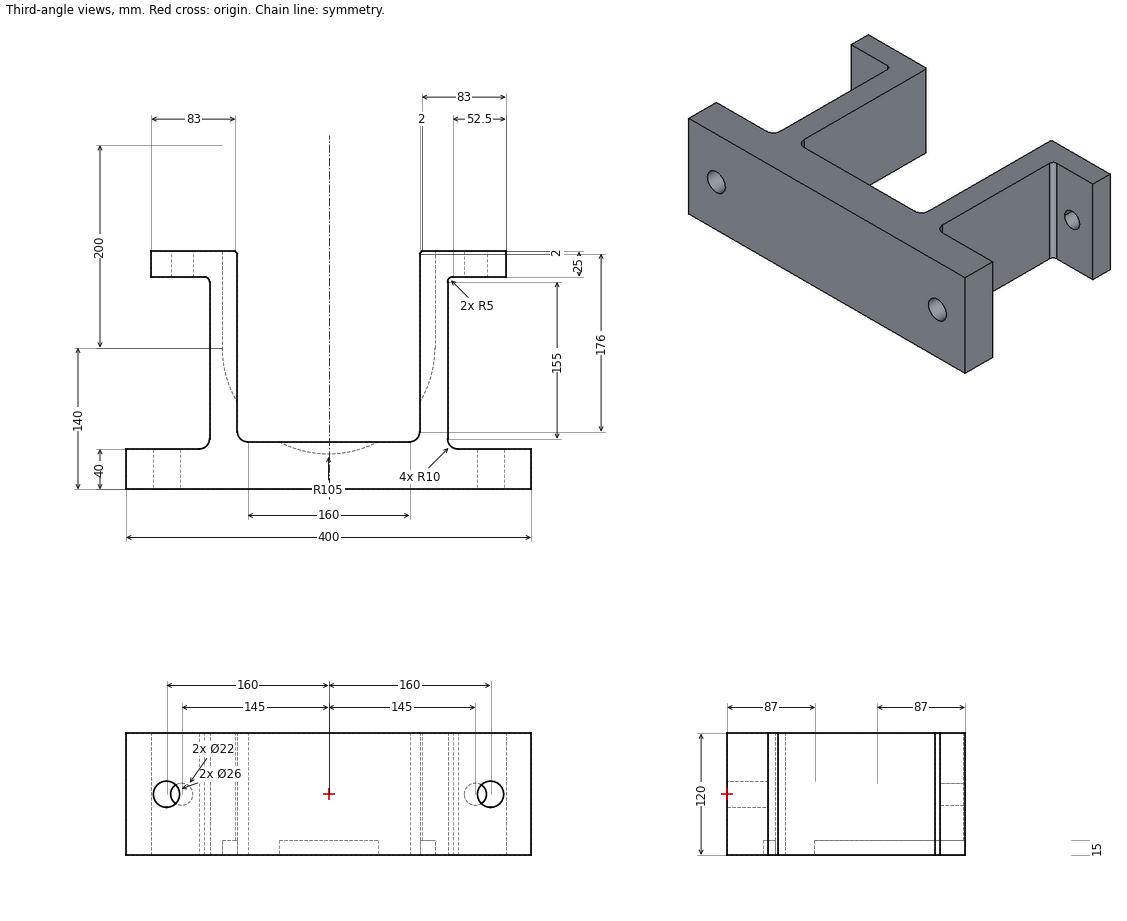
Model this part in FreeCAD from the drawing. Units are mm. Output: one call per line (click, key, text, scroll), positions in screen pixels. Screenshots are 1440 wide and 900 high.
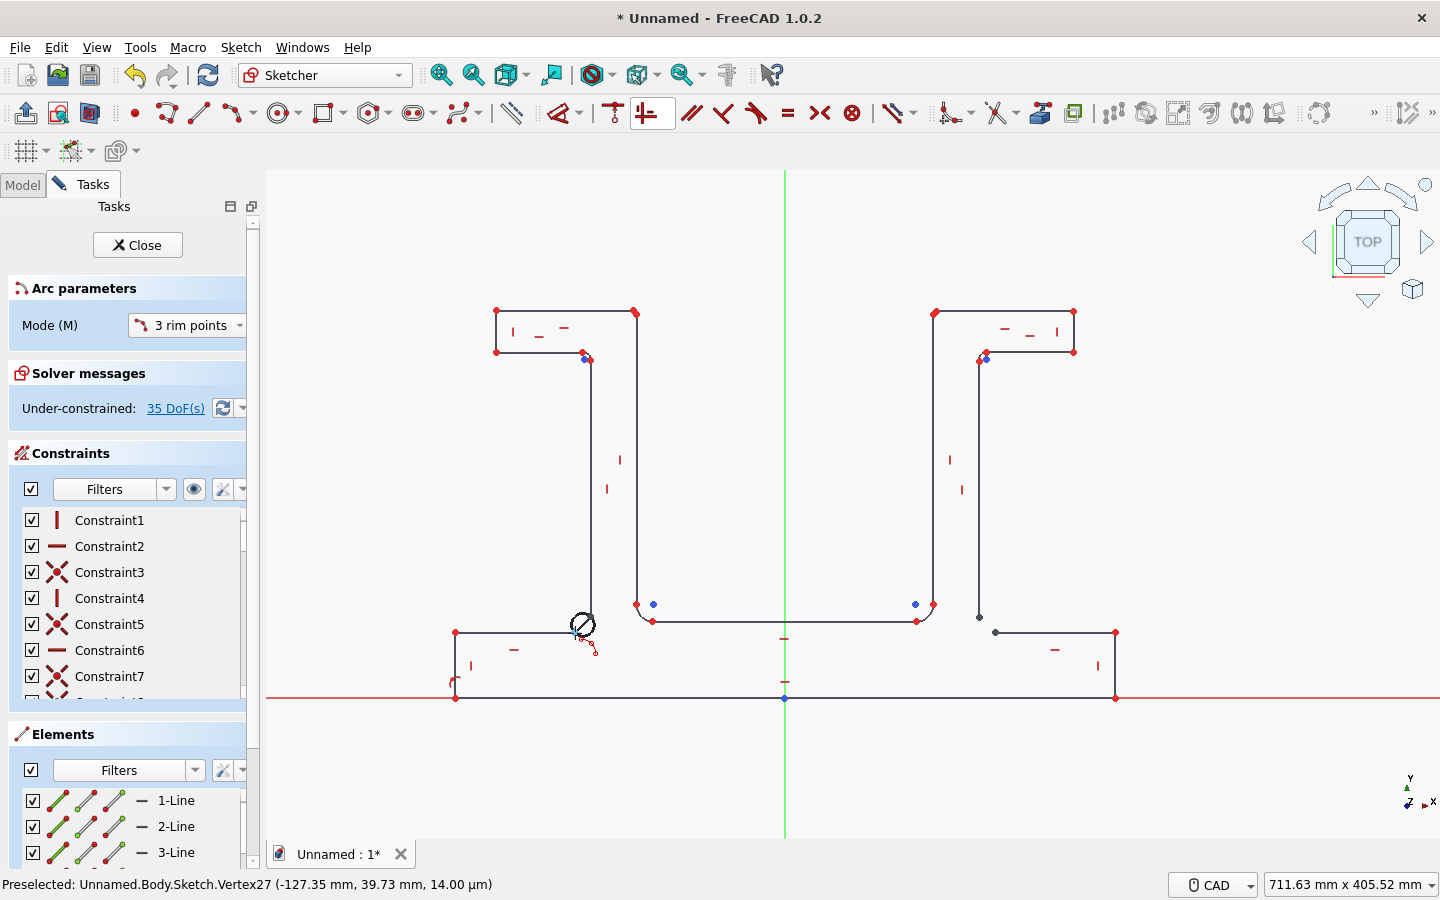
scroll(586, 628, up, 6)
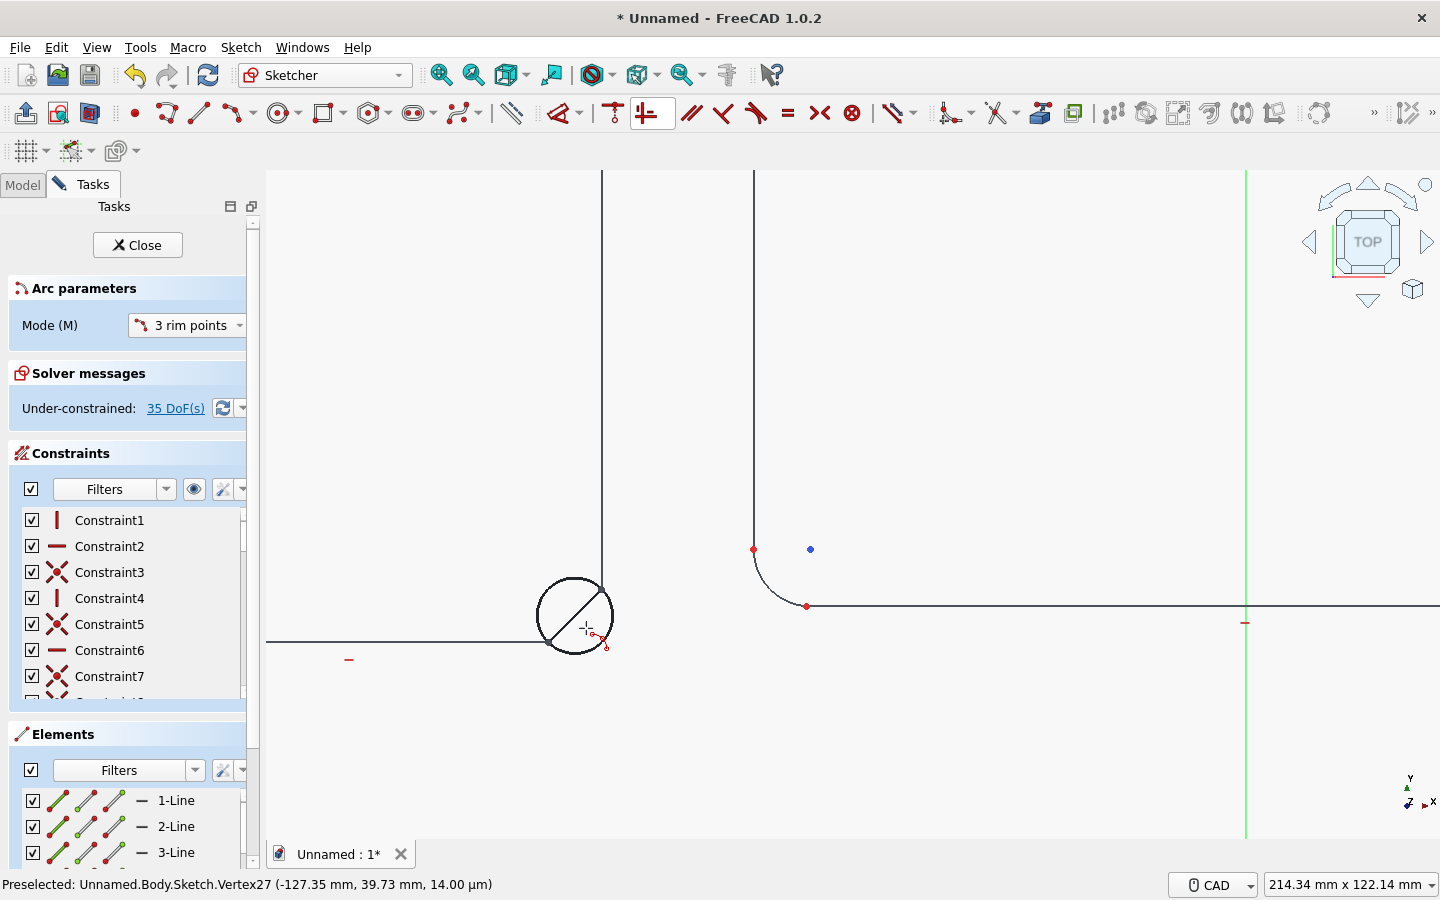
click(586, 625)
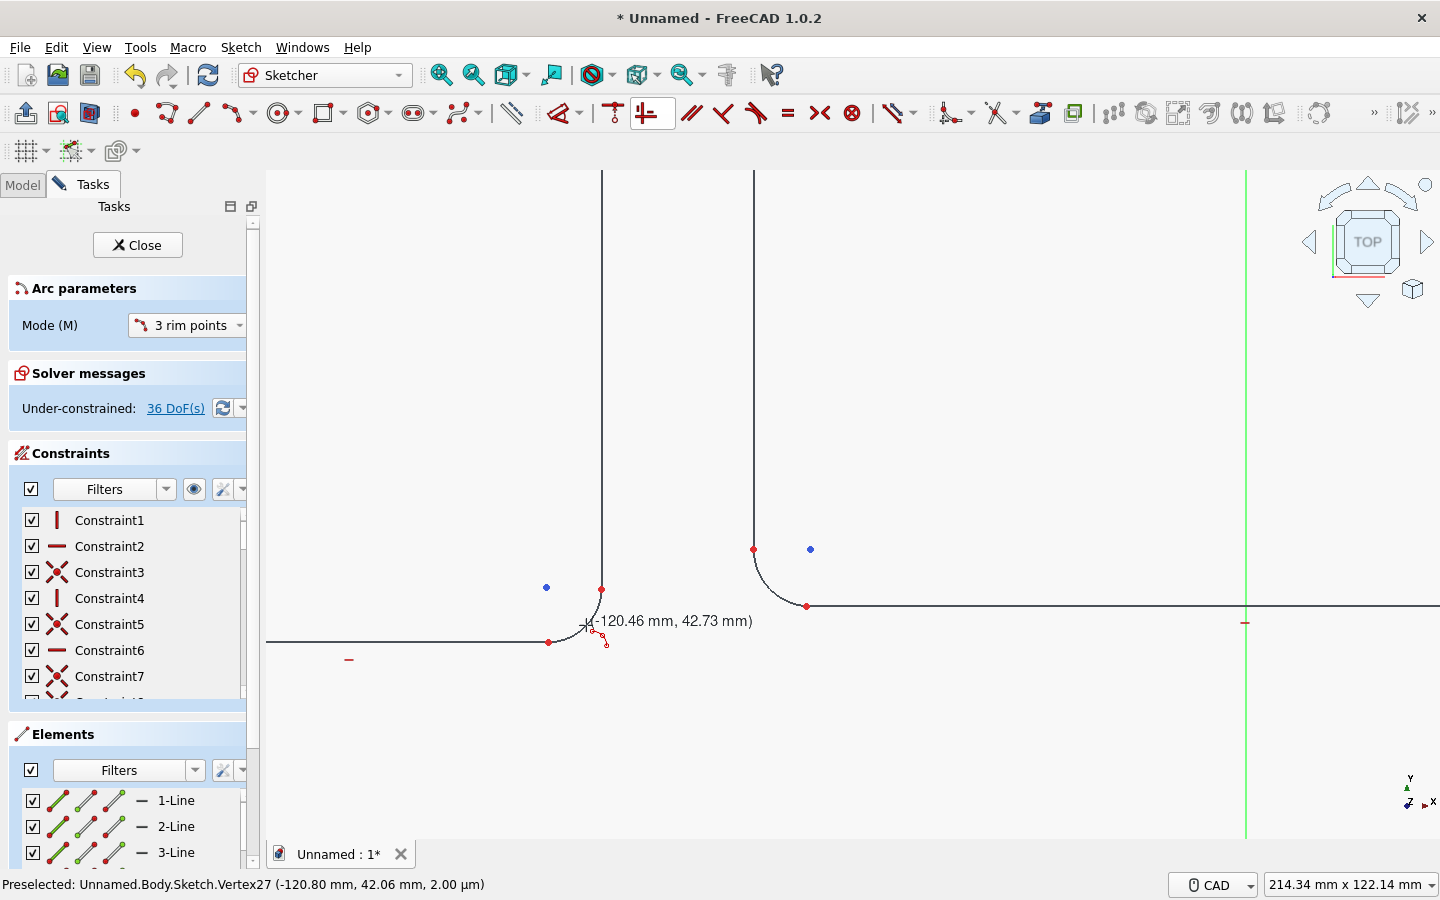
scroll(586, 629, down, 6)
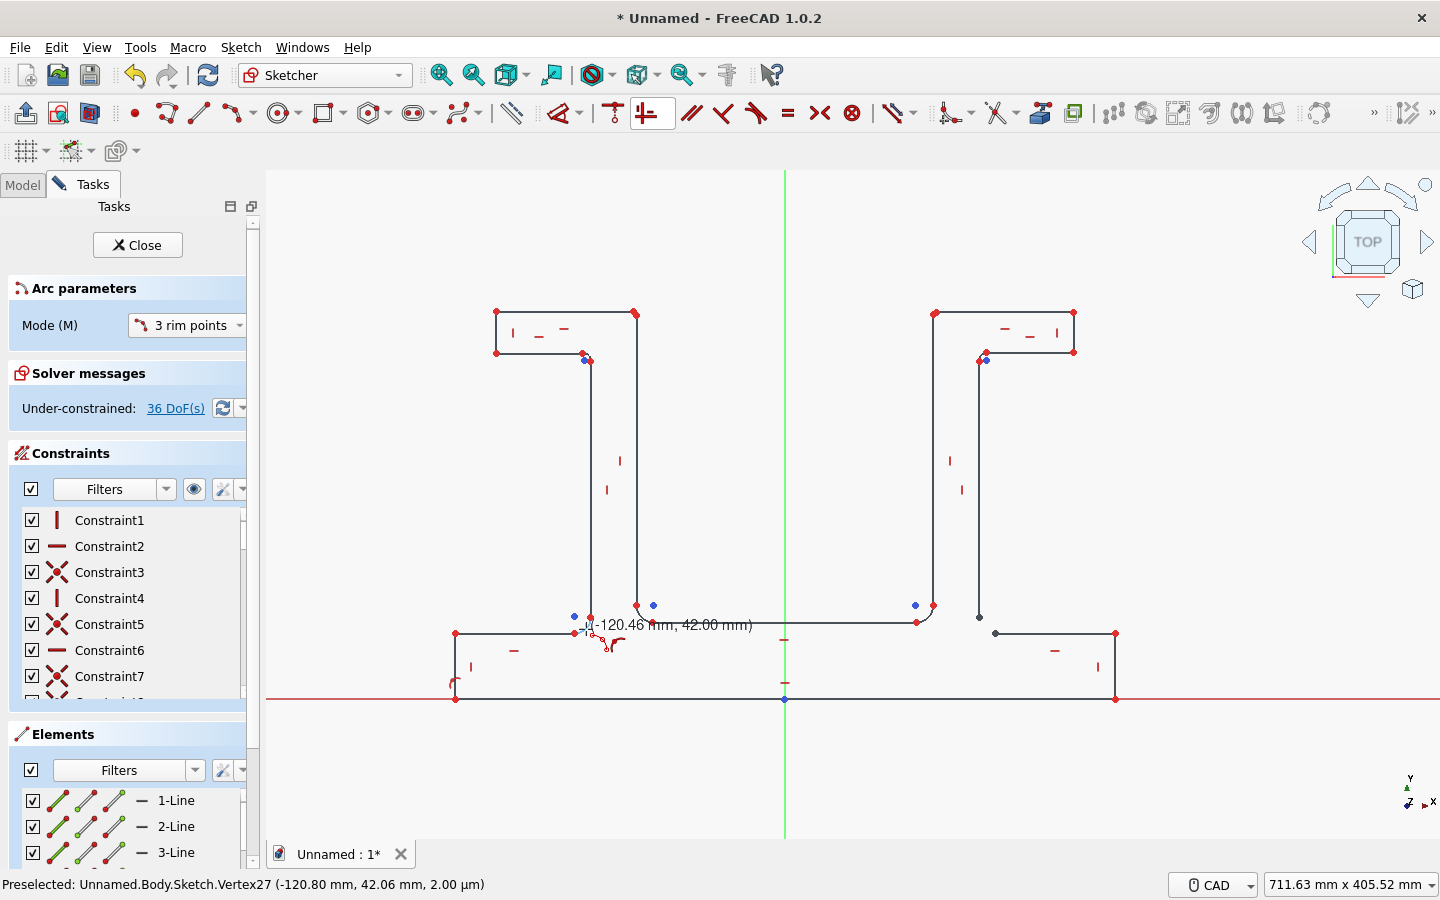
click(995, 634)
click(979, 618)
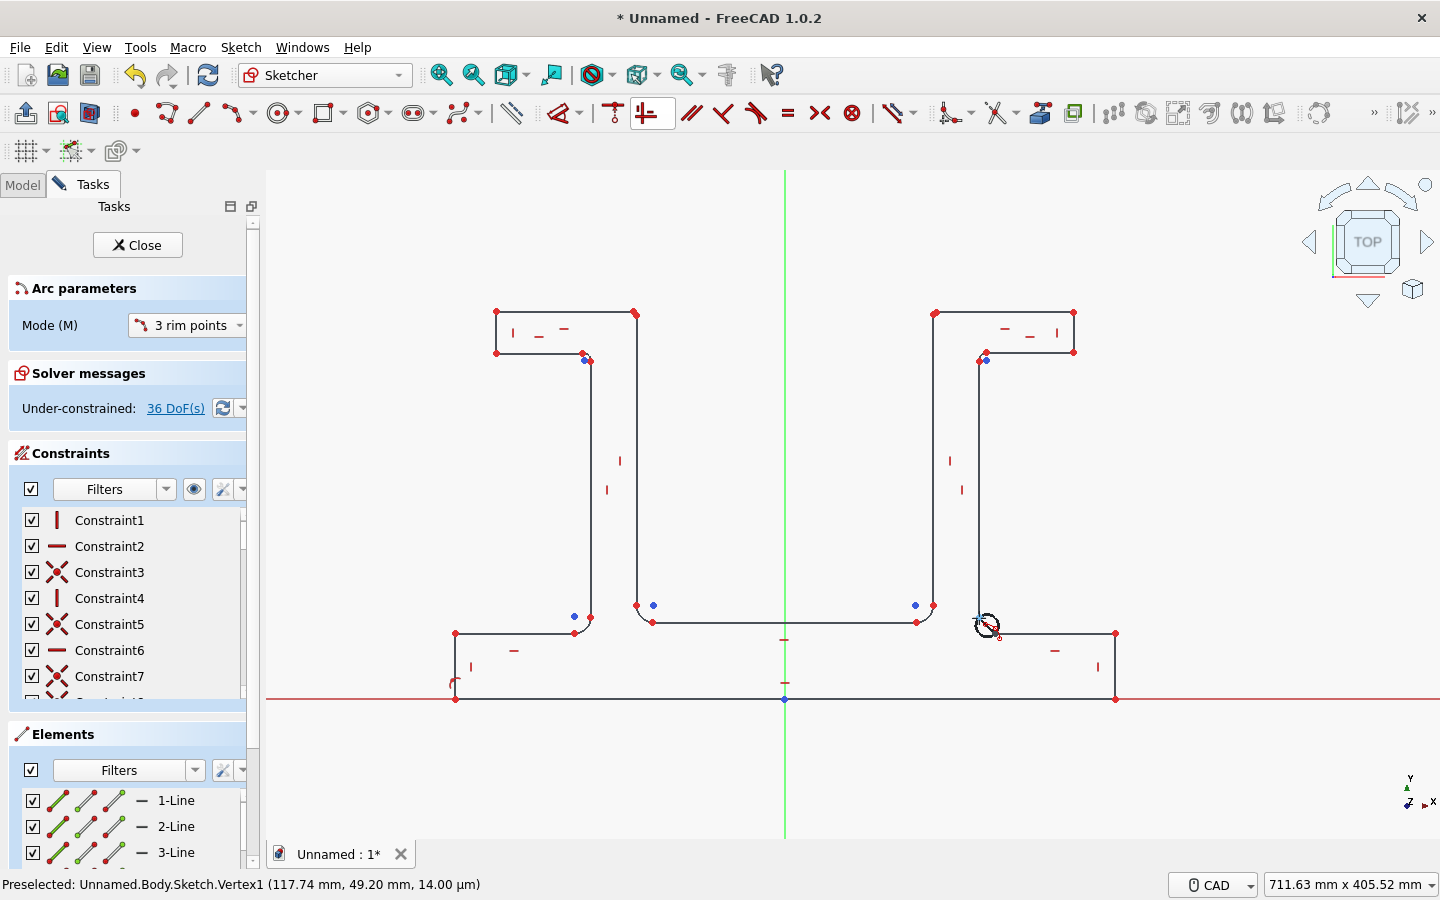
scroll(984, 628, up, 6)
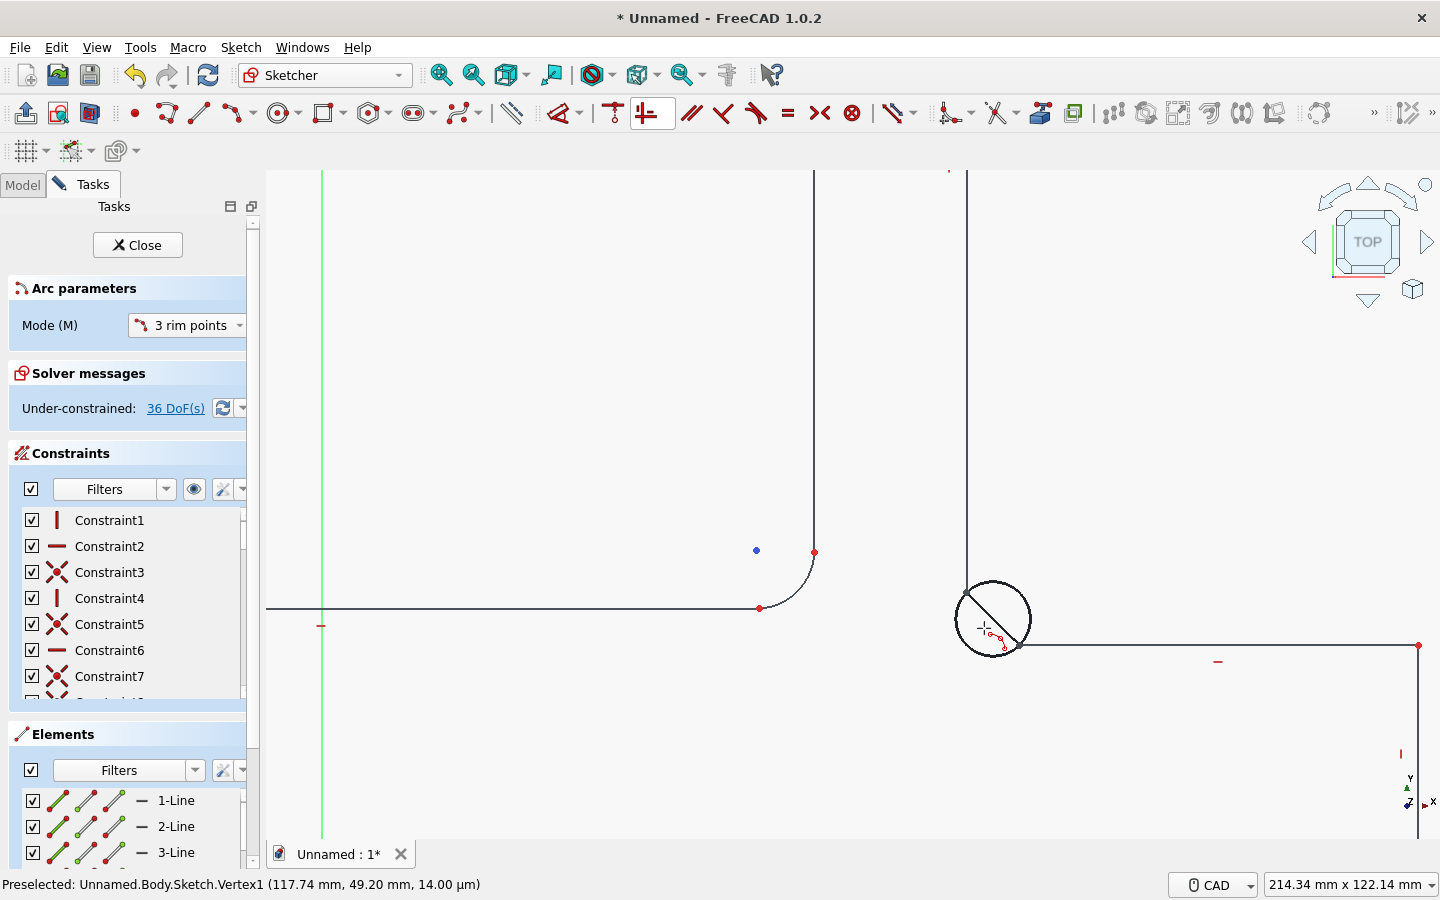
click(981, 627)
key(Escape)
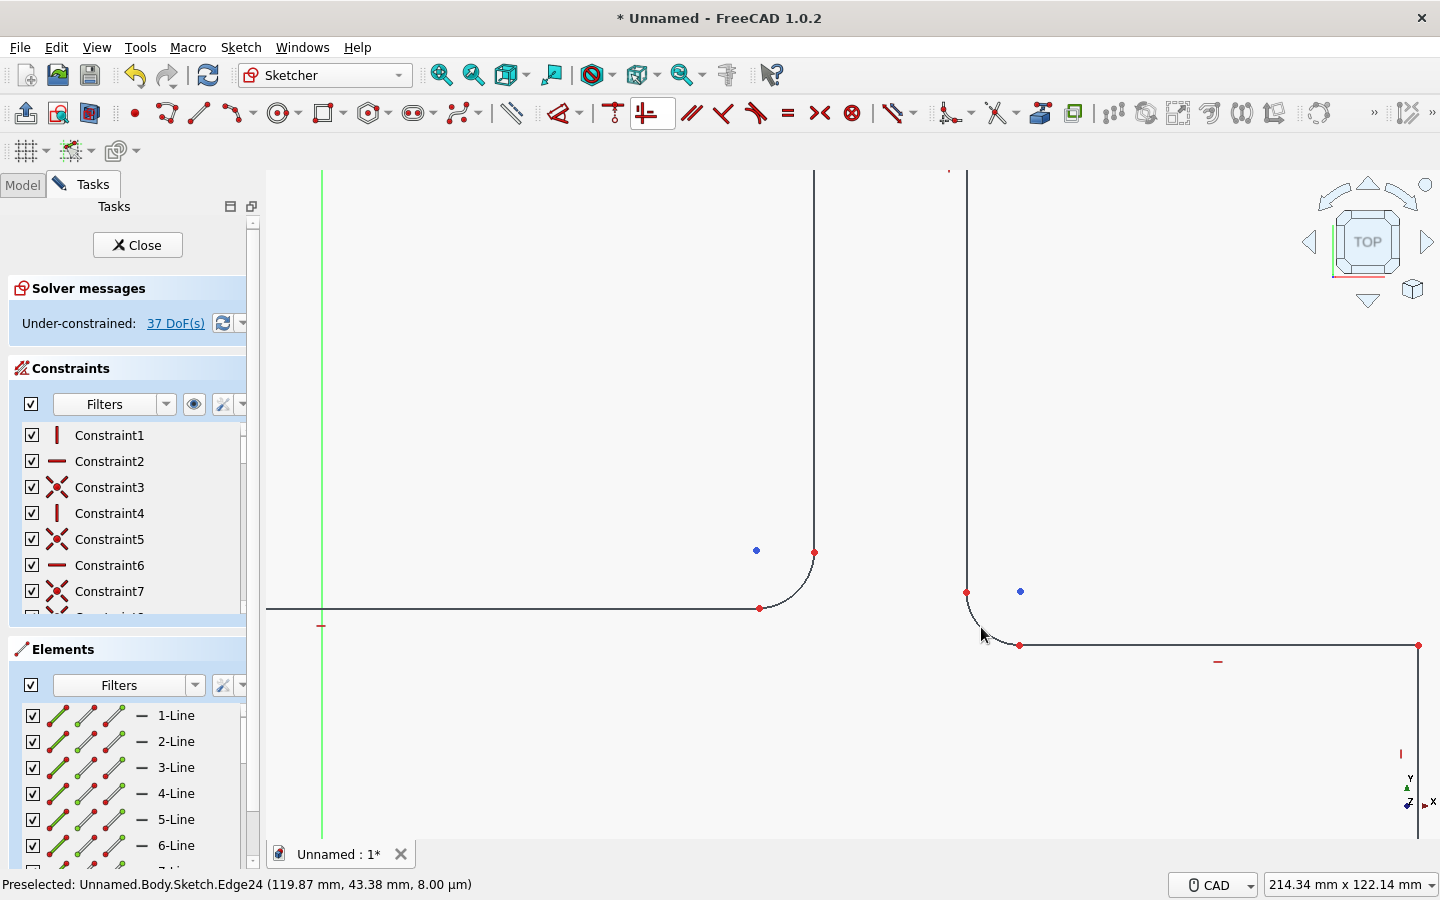
click(967, 338)